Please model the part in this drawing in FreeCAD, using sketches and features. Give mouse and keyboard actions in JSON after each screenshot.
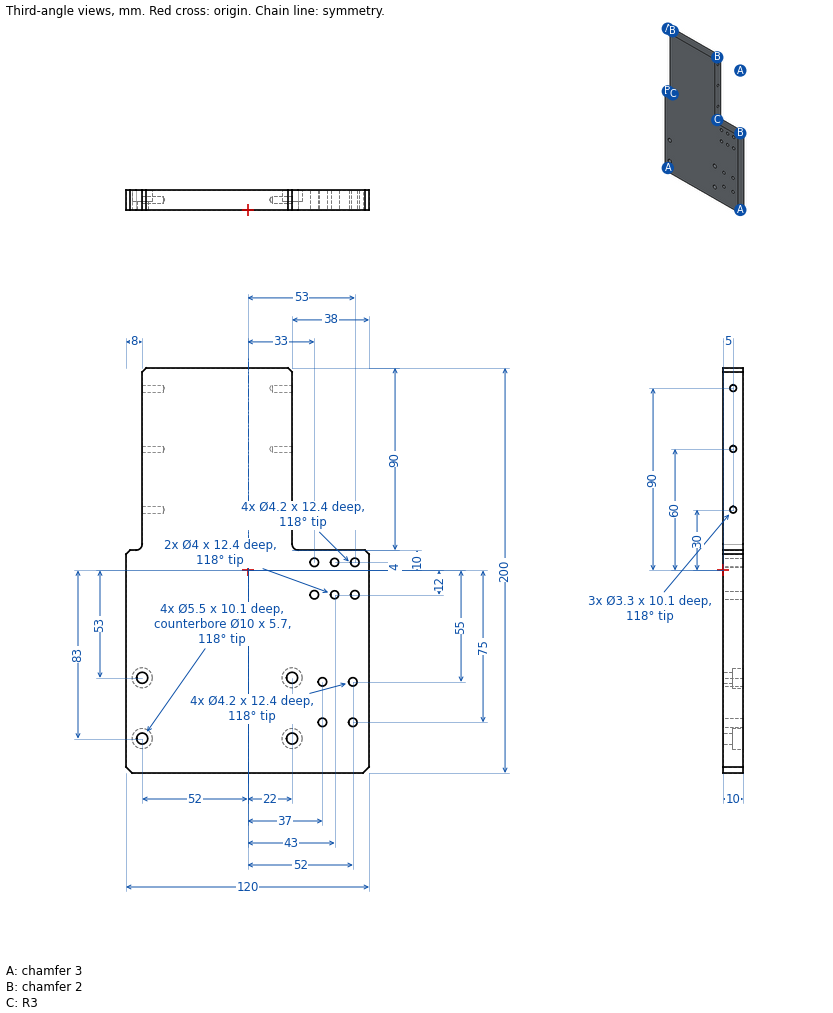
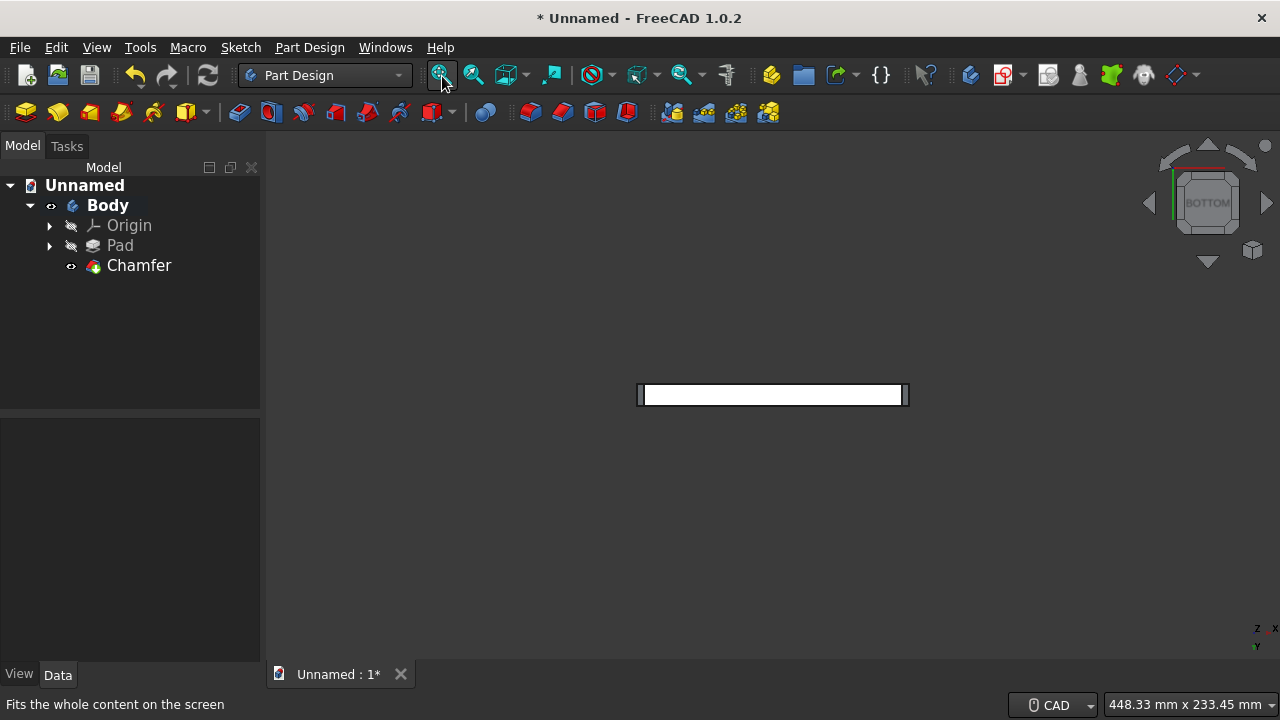
{"action": "key", "text": "4"}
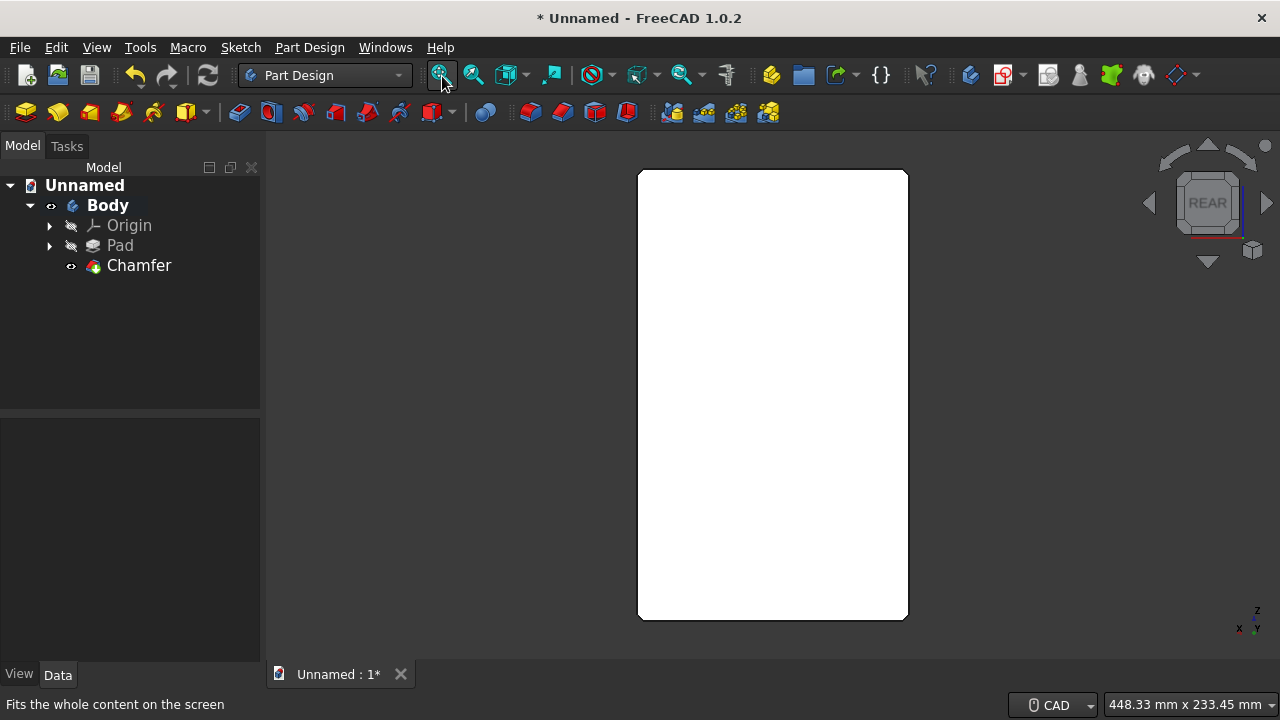
{"action": "left_click", "coordinate": [773, 329]}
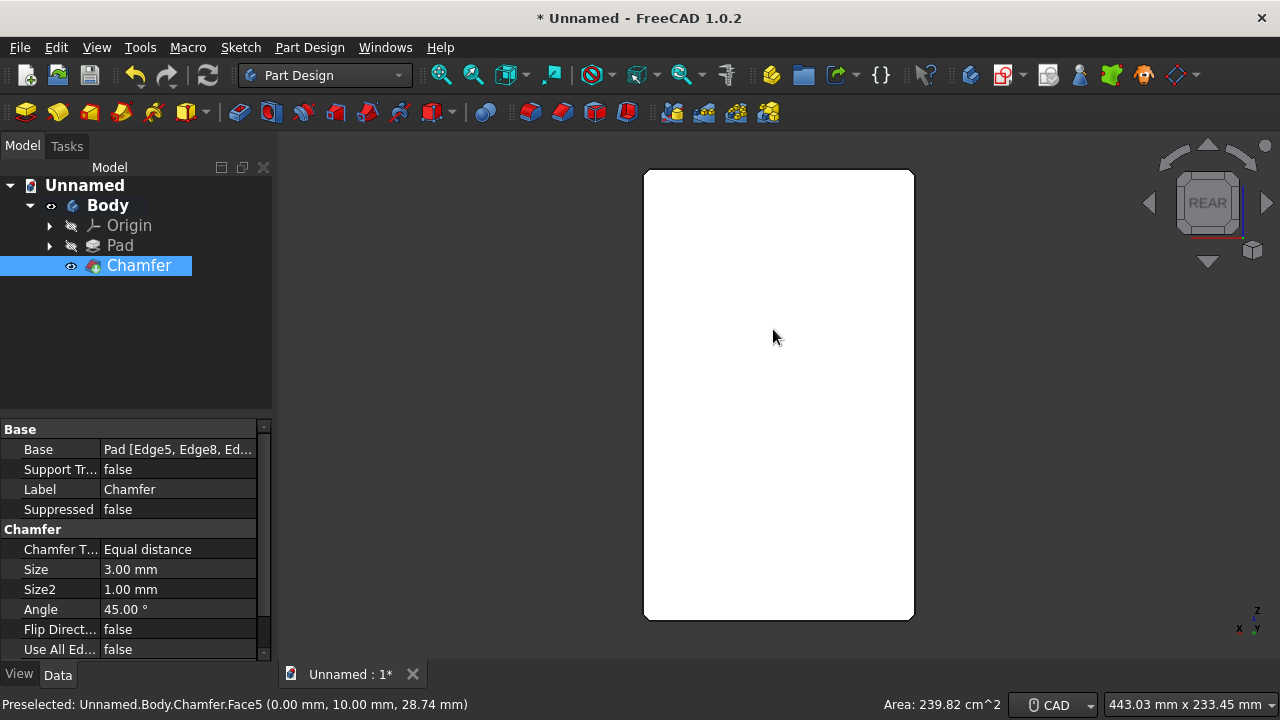
{"action": "left_click", "coordinate": [1004, 76]}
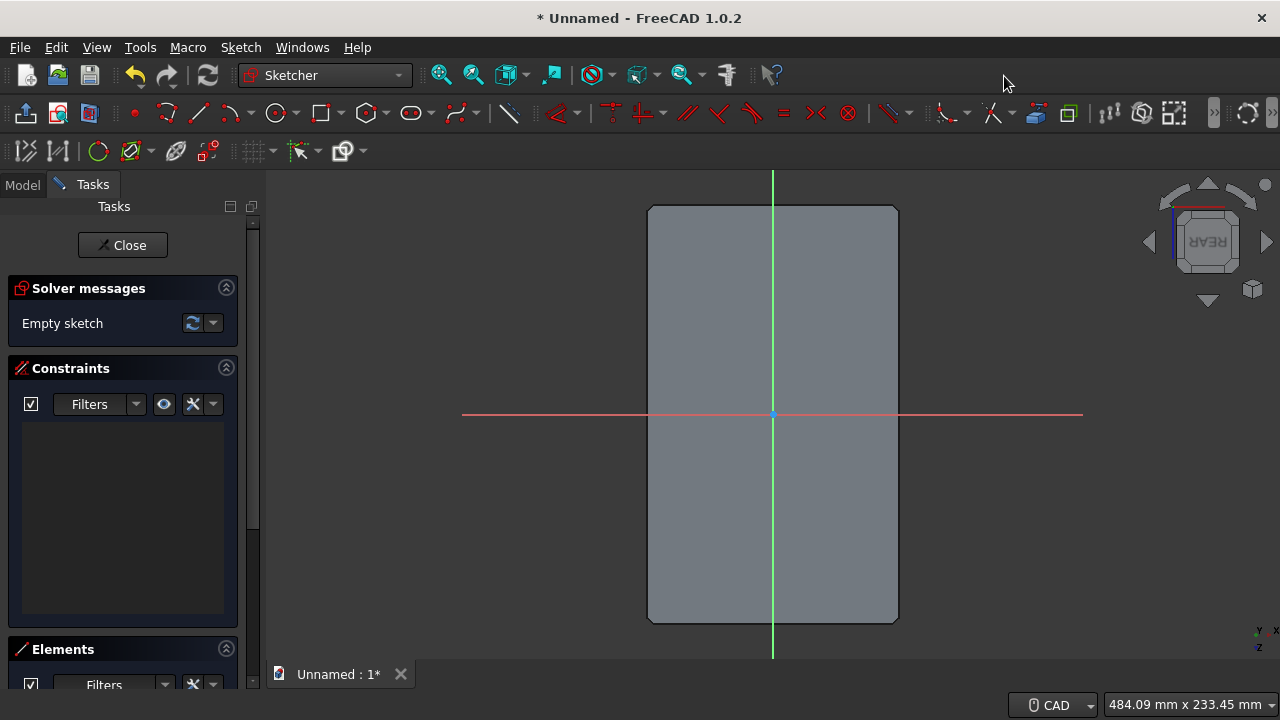
{"action": "scroll", "coordinate": [787, 215], "scroll_direction": "up", "scroll_amount": 3}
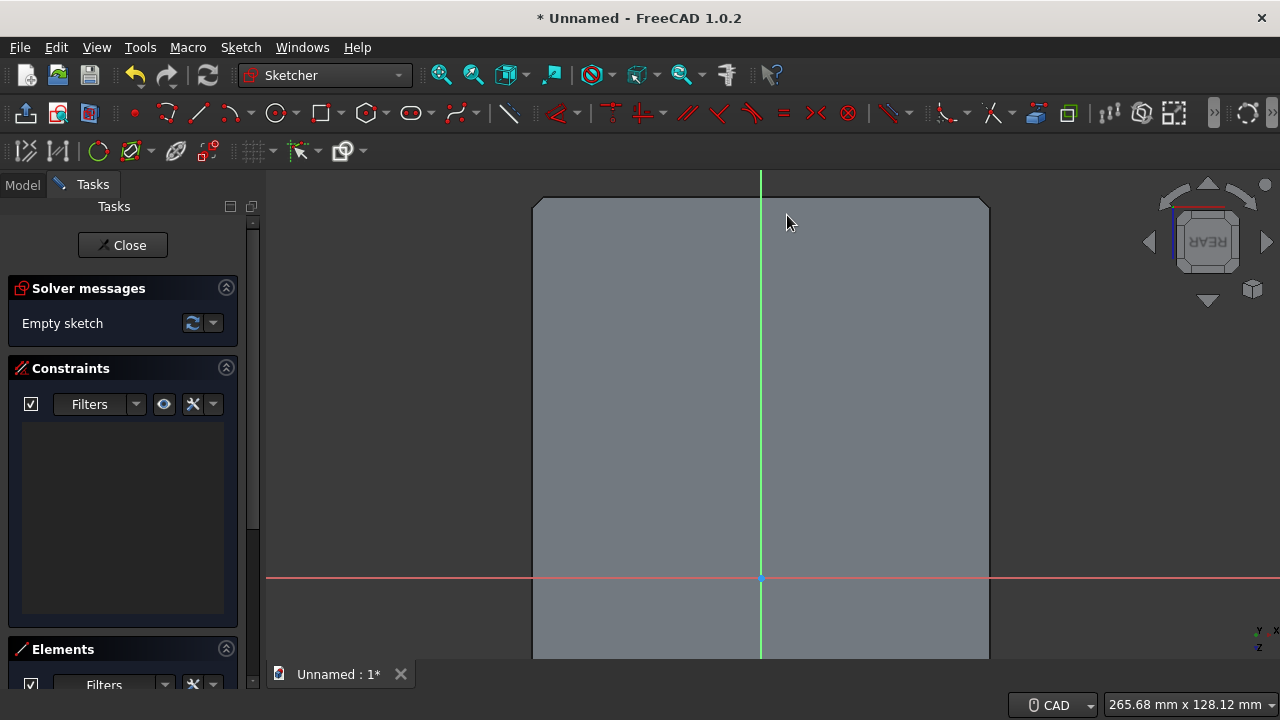
{"action": "left_click", "coordinate": [276, 114]}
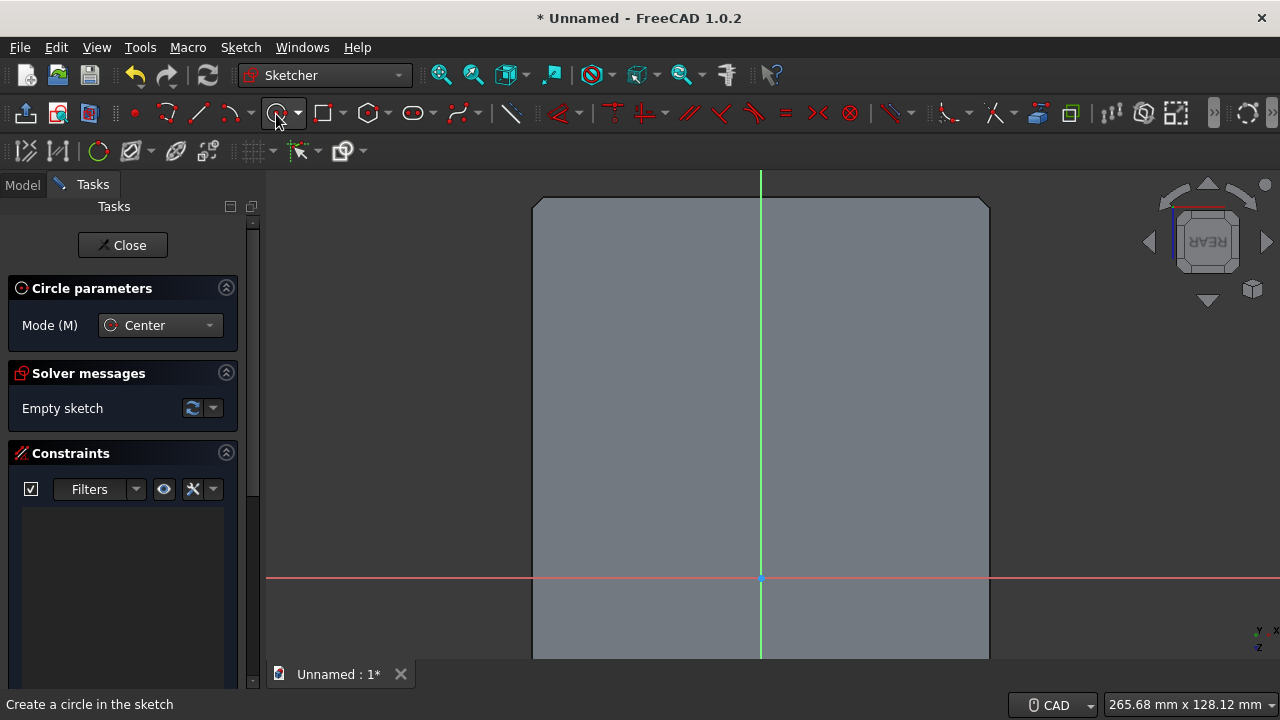
{"action": "scroll", "coordinate": [563, 262], "scroll_direction": "up", "scroll_amount": 4}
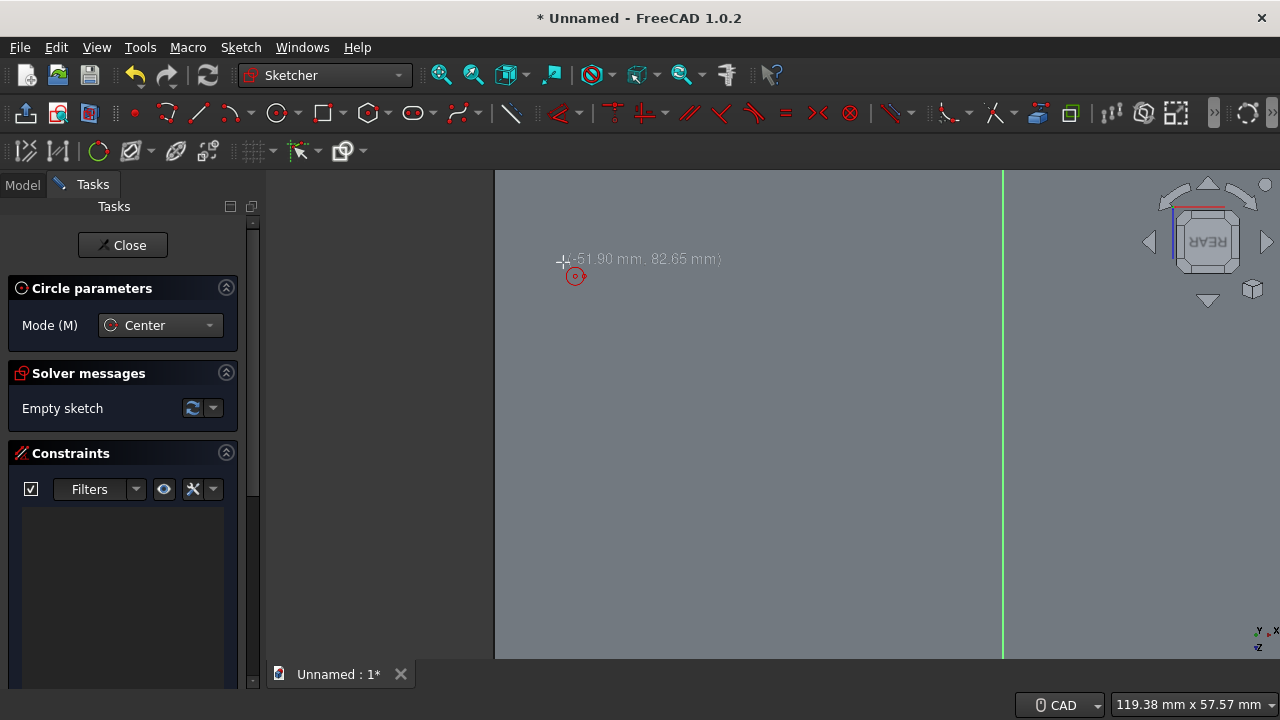
{"action": "left_click", "coordinate": [562, 261]}
{"action": "left_click", "coordinate": [578, 244]}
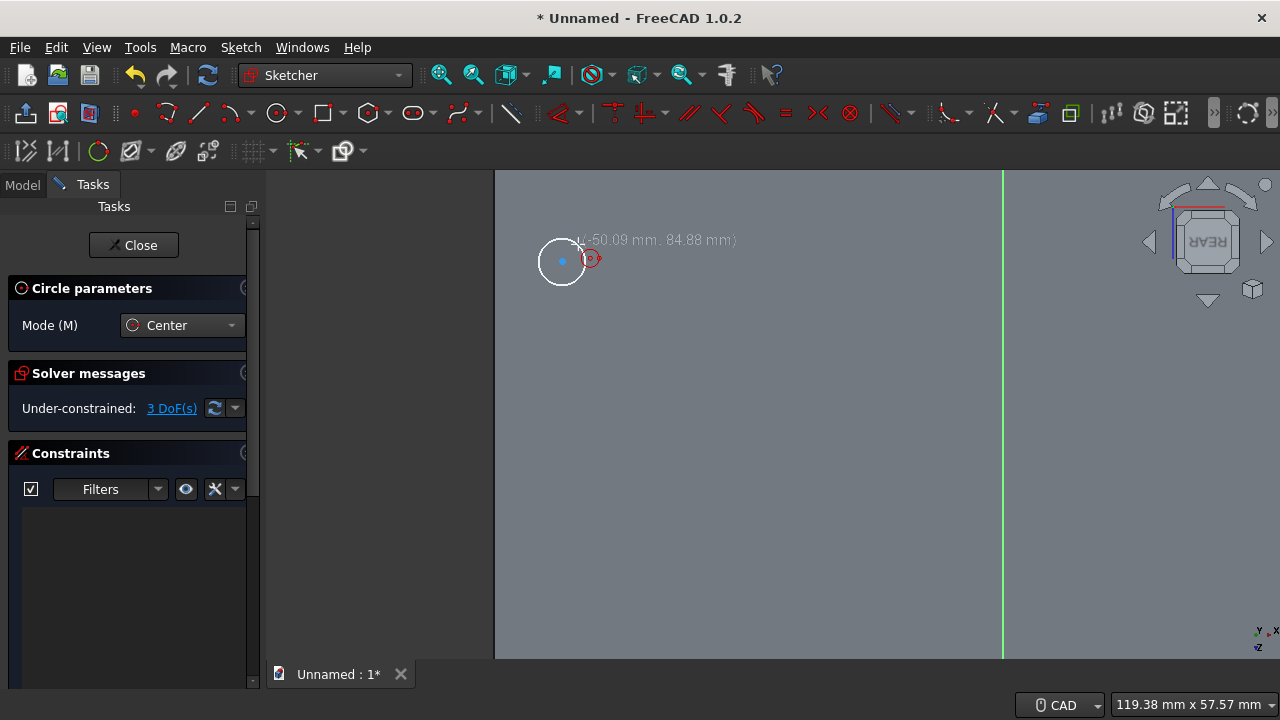
{"action": "left_click", "coordinate": [562, 516]}
{"action": "left_click", "coordinate": [578, 499]}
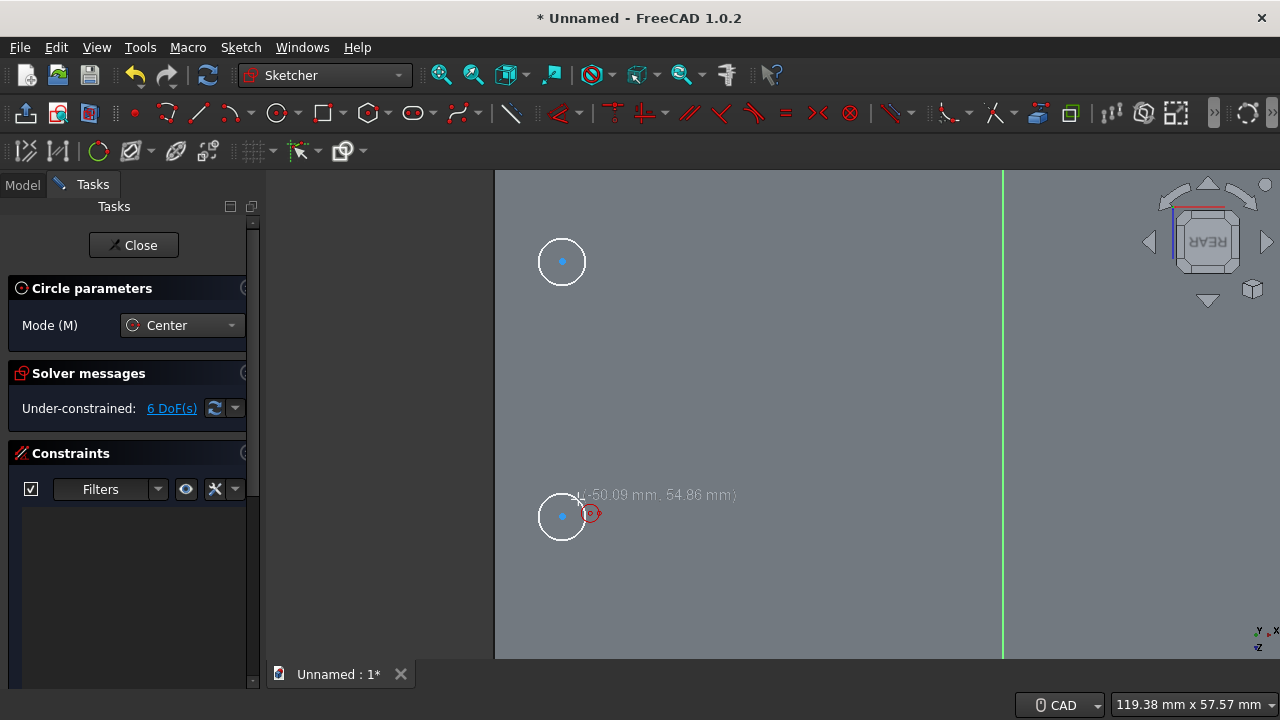
{"action": "scroll", "coordinate": [565, 262], "scroll_direction": "down", "scroll_amount": 4}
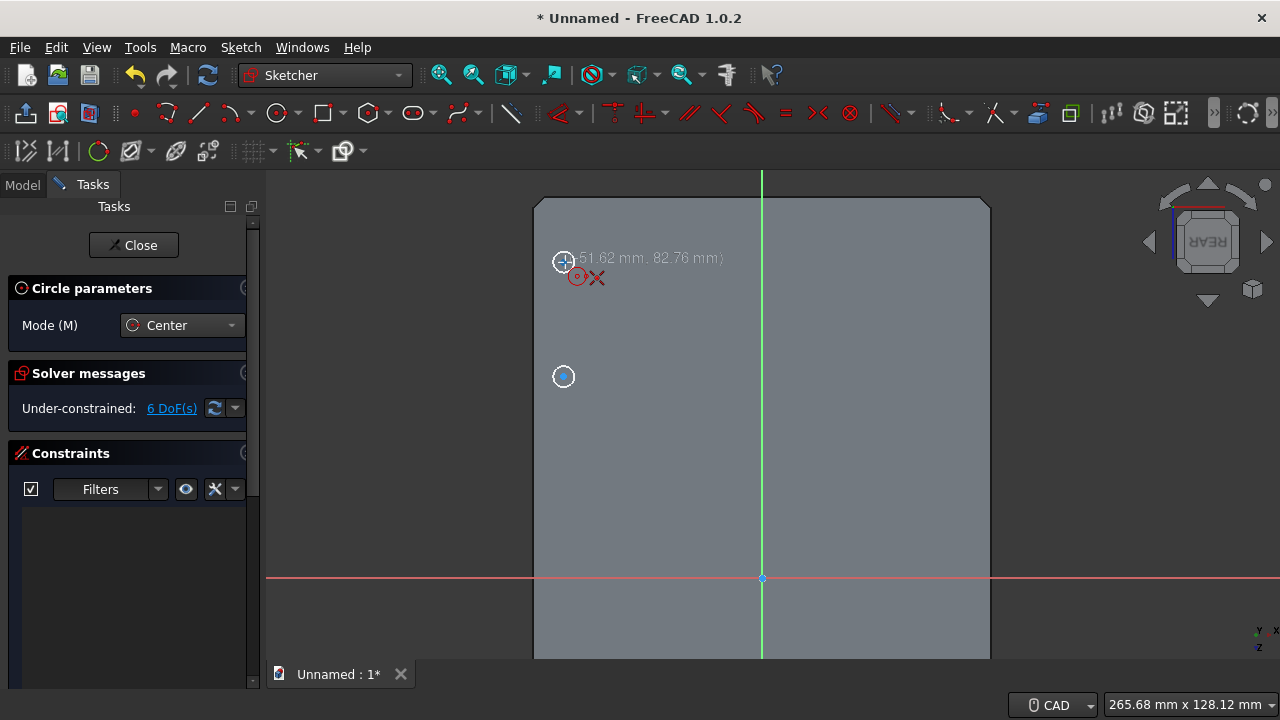
{"action": "scroll", "coordinate": [846, 376], "scroll_direction": "up", "scroll_amount": 4}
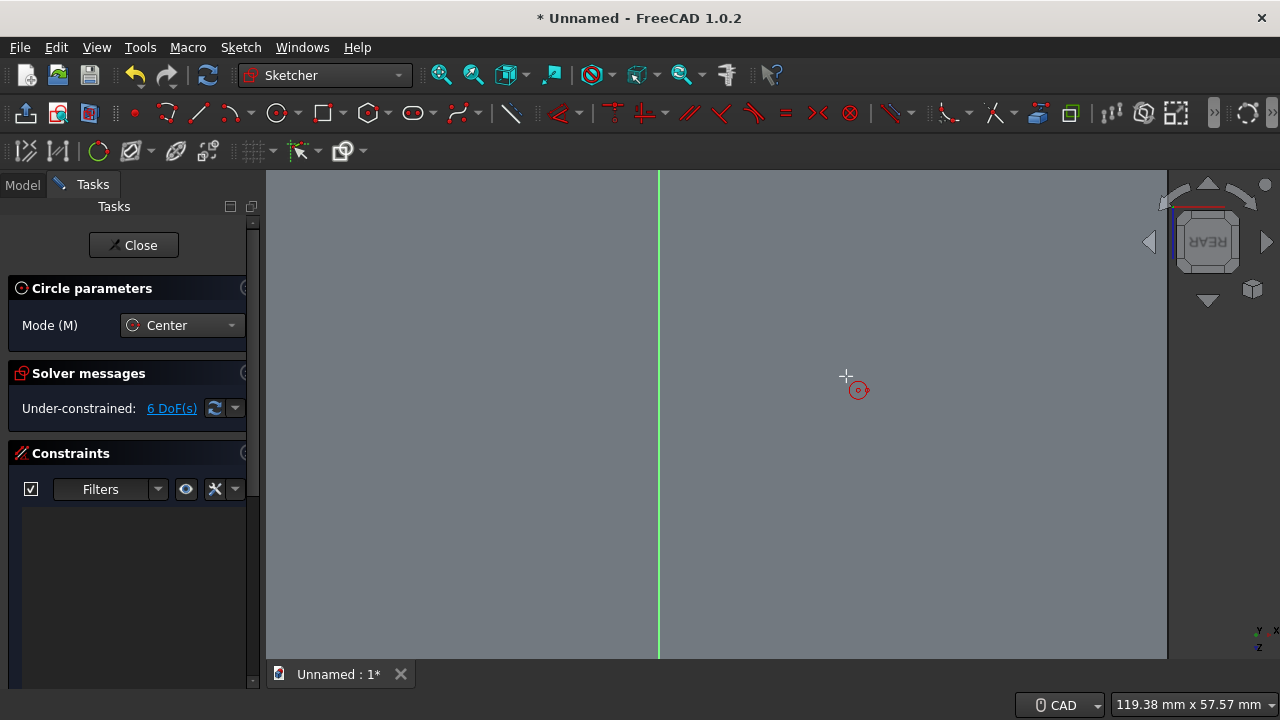
{"action": "left_click", "coordinate": [846, 376]}
{"action": "left_click", "coordinate": [862, 359]}